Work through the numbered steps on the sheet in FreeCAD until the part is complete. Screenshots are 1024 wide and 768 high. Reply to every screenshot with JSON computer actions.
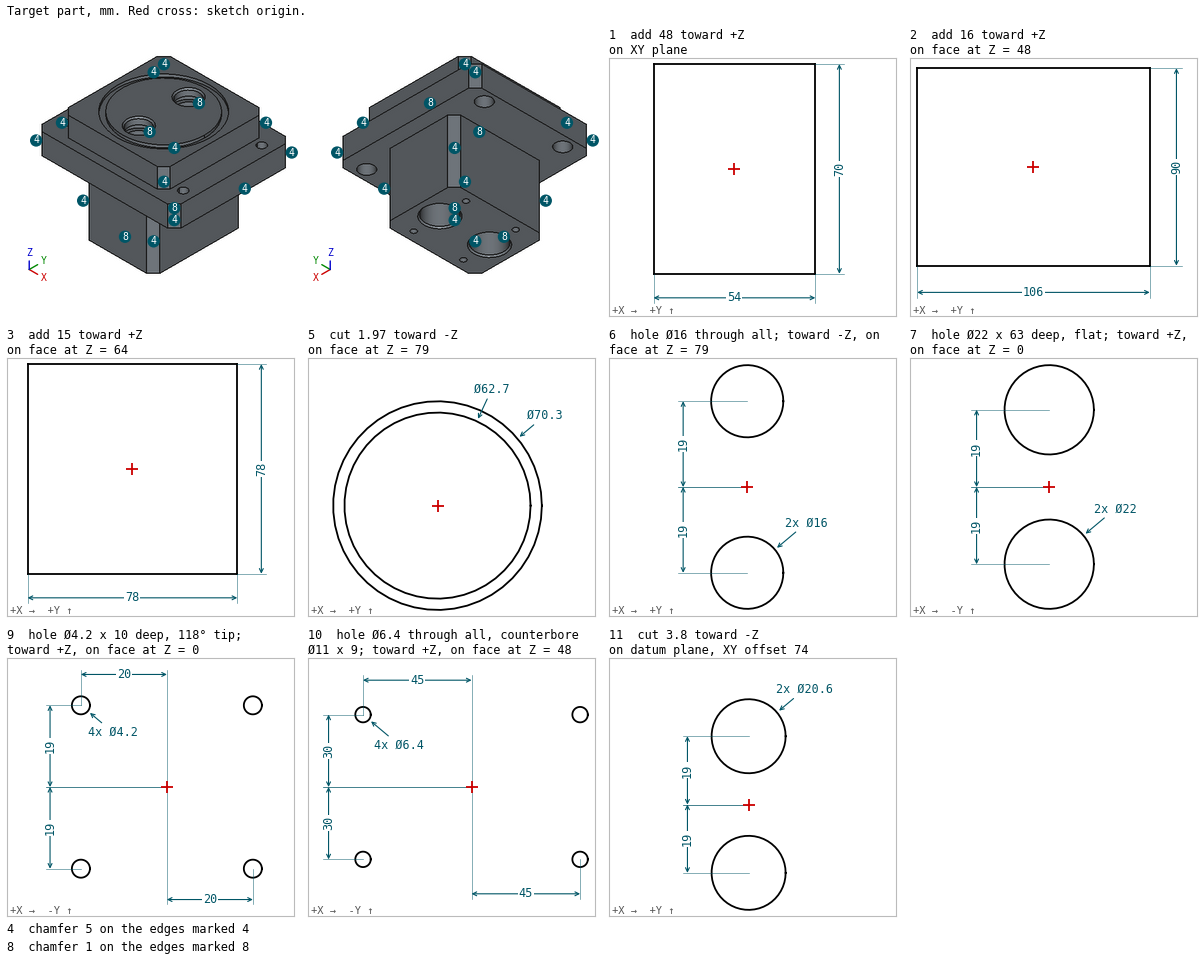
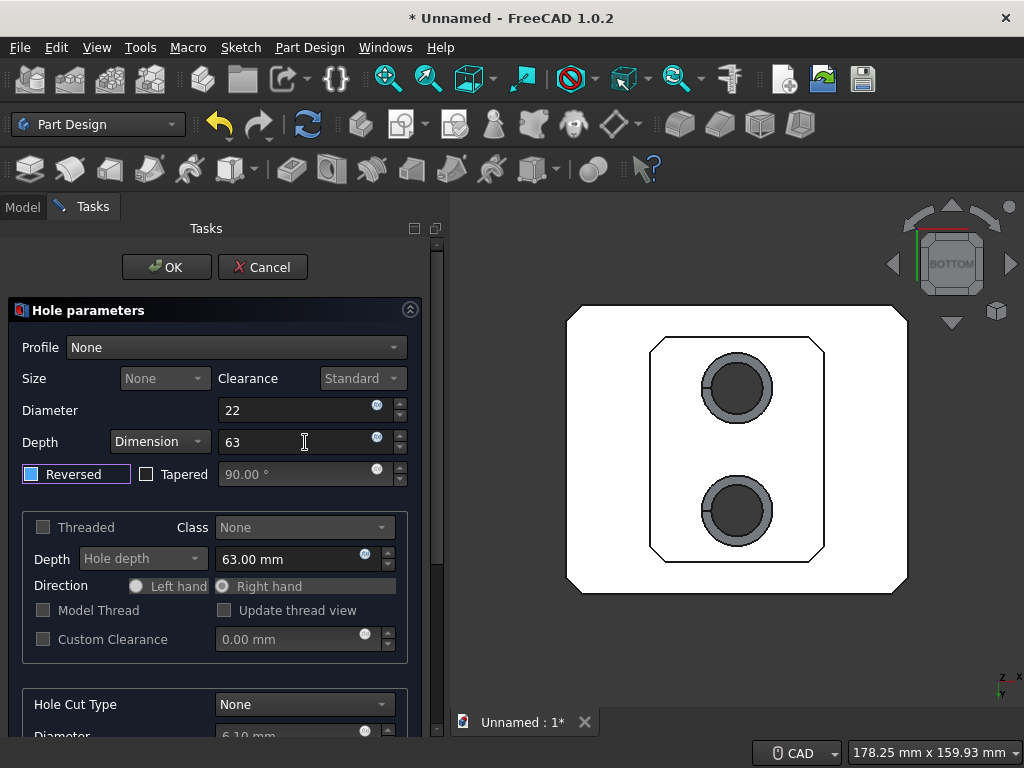
{"action": "scroll", "coordinate": [437, 487], "scroll_direction": "down", "scroll_amount": 4}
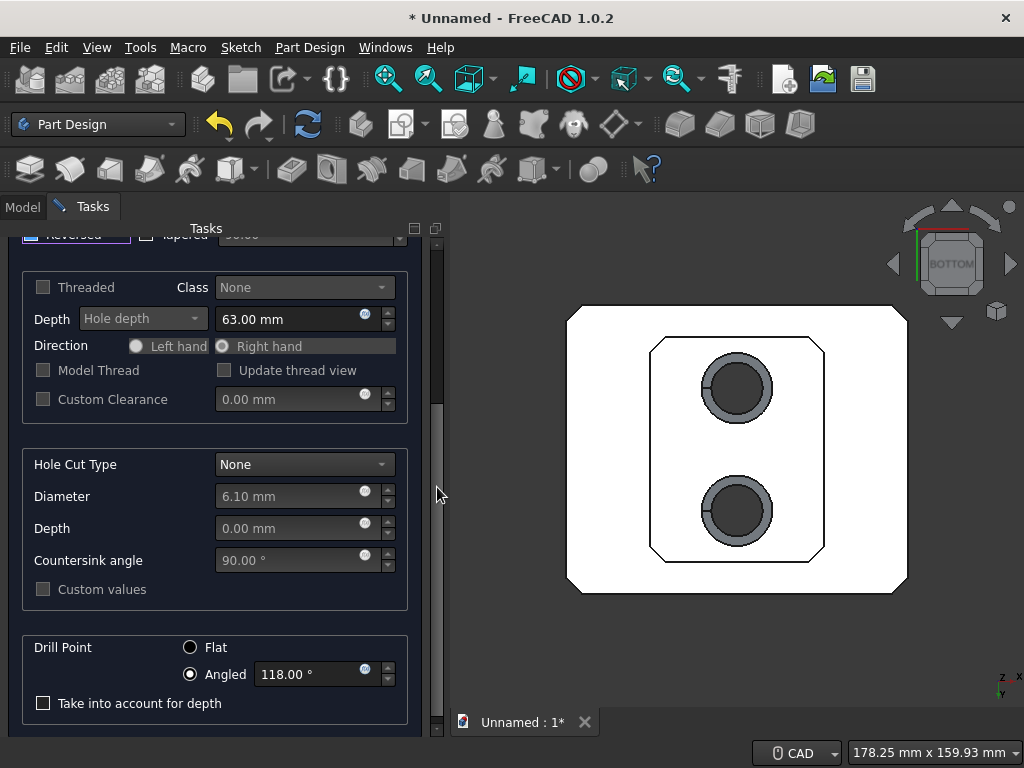
{"action": "left_click", "coordinate": [191, 647]}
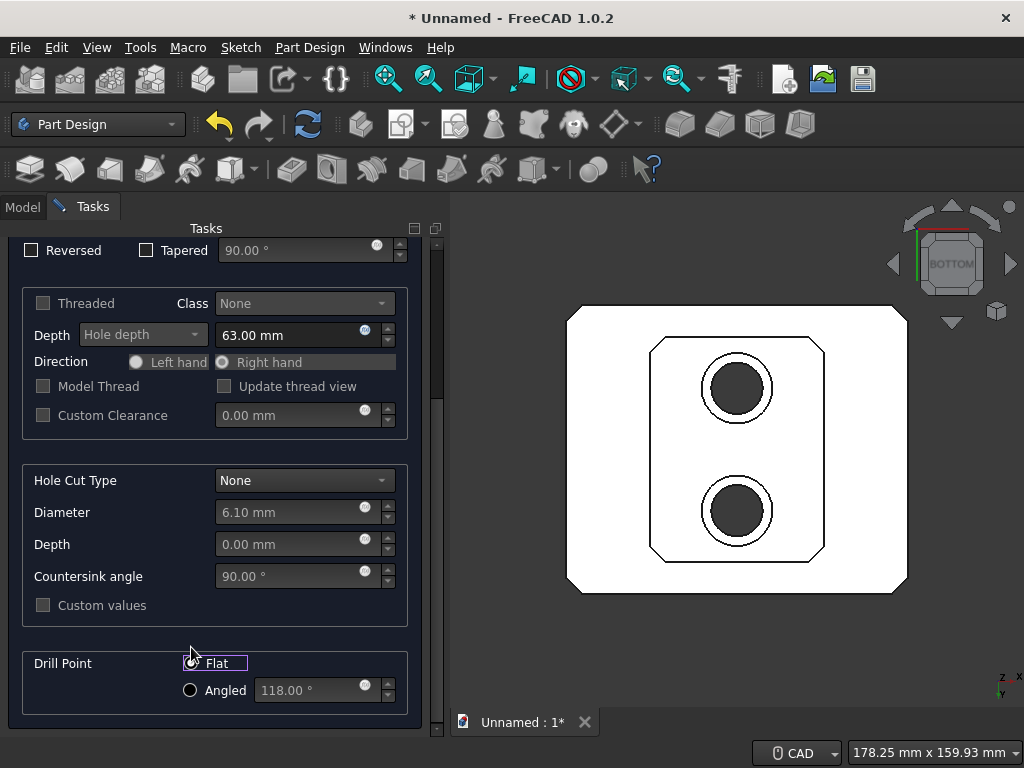
{"action": "scroll", "coordinate": [437, 487], "scroll_direction": "up", "scroll_amount": 5}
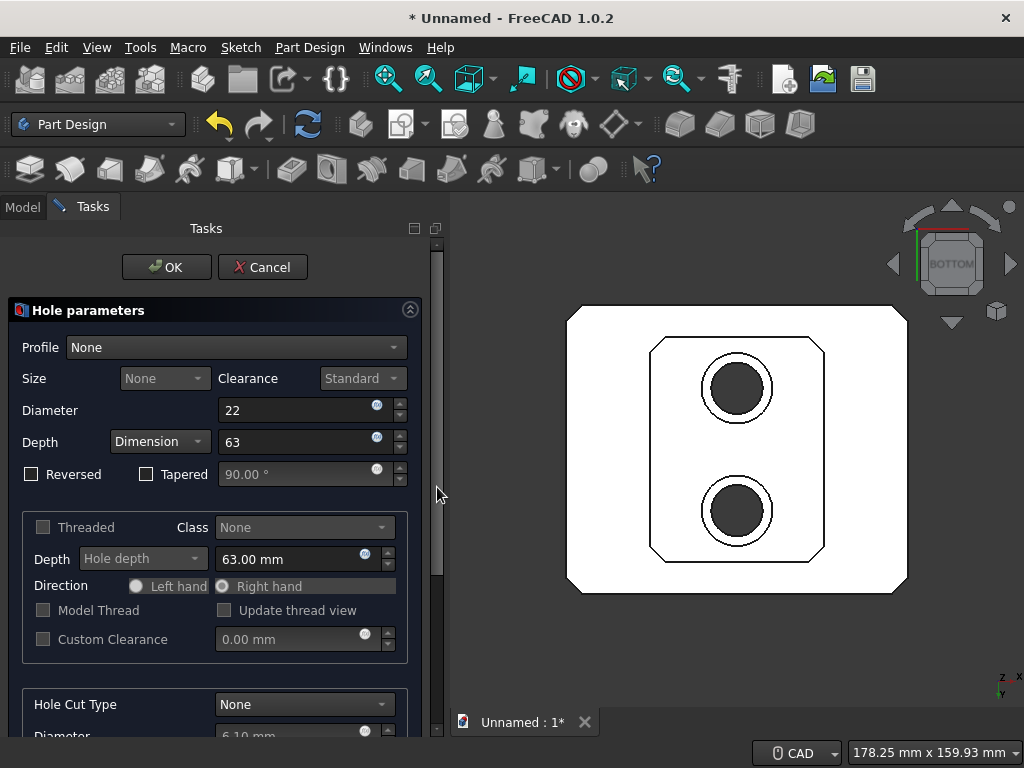
{"action": "left_click", "coordinate": [167, 267]}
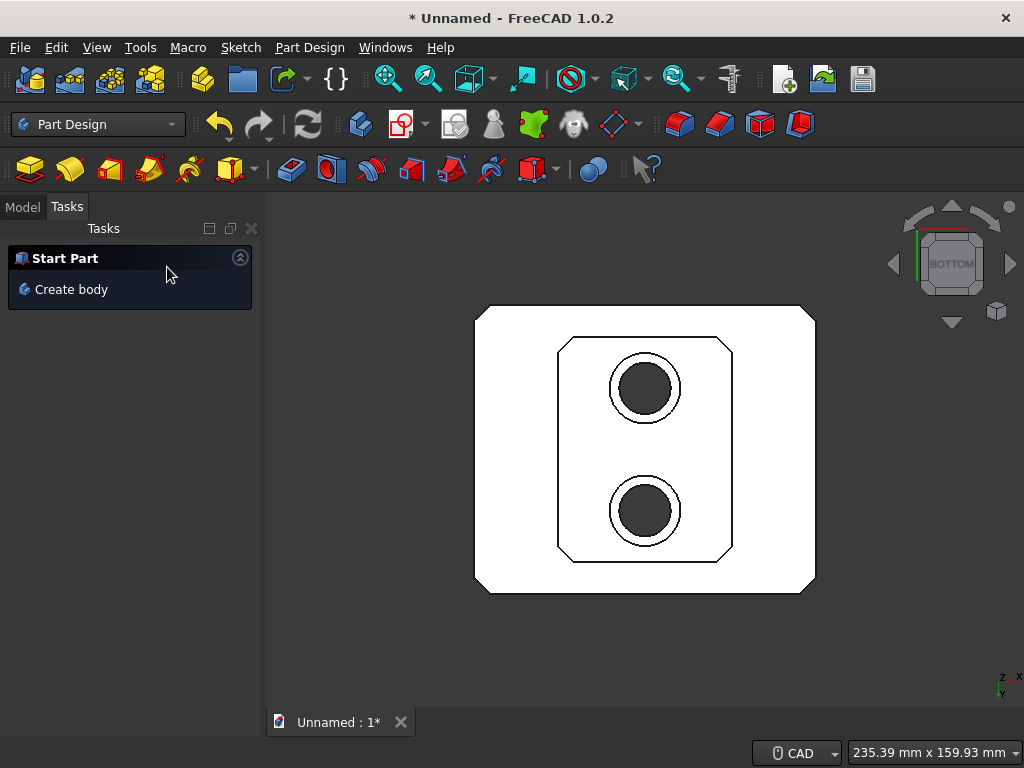
{"action": "left_click", "coordinate": [674, 366]}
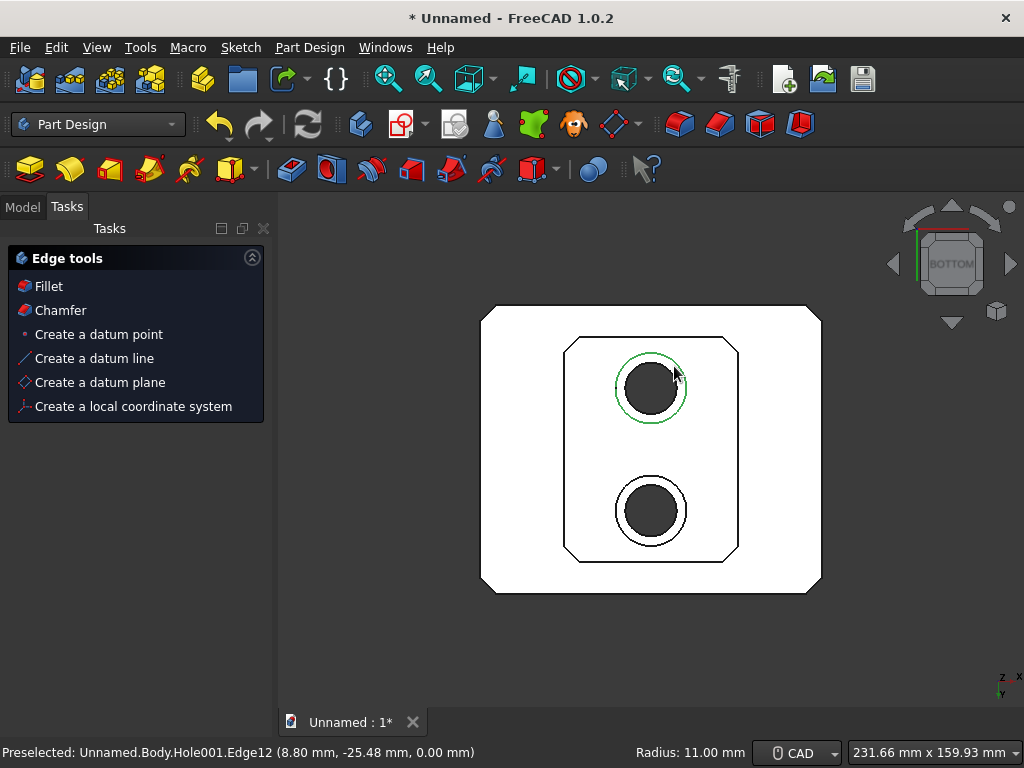
{"action": "left_click", "coordinate": [680, 531], "text": "ctrl"}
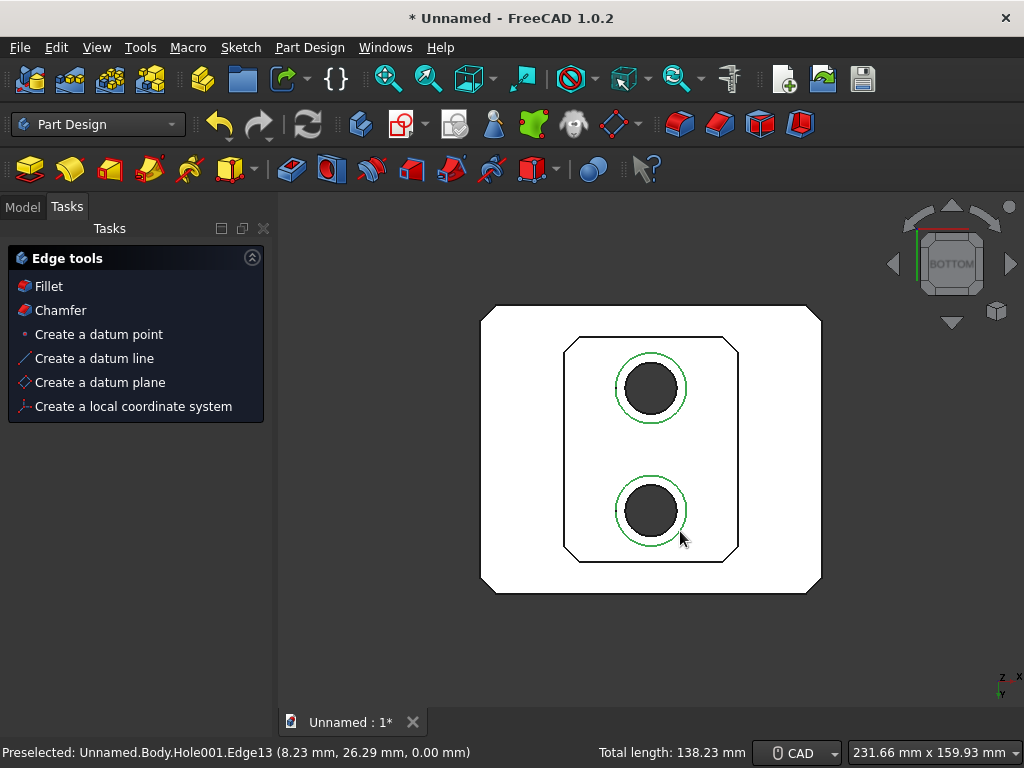
{"action": "key", "text": "0"}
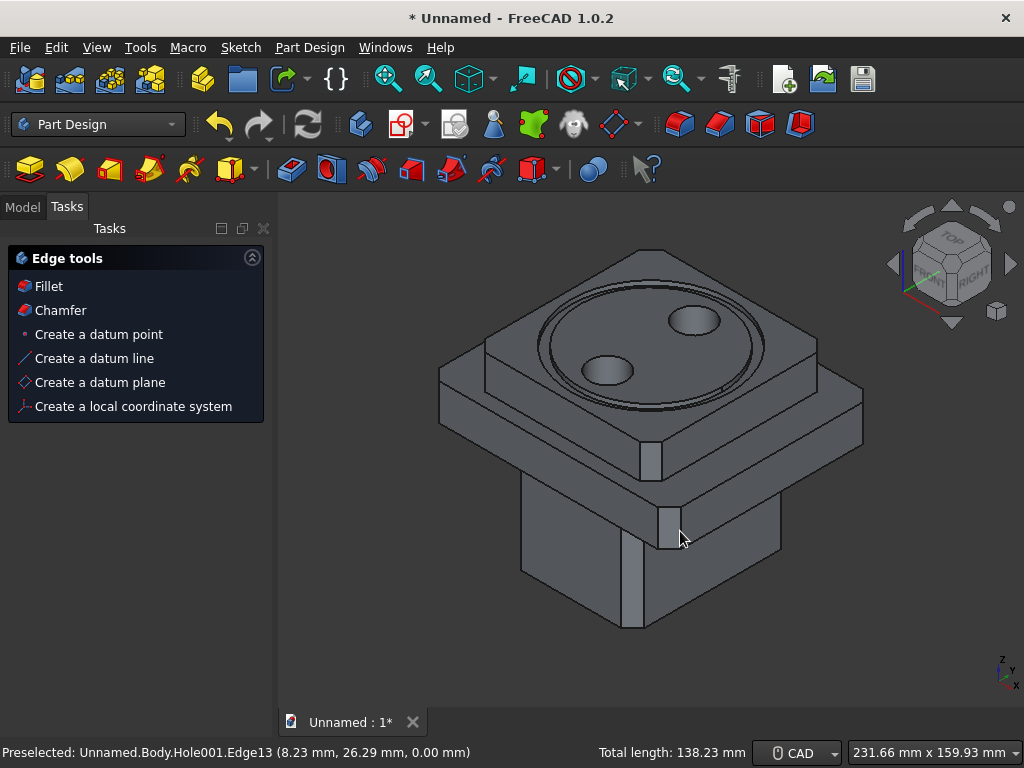
{"action": "left_click", "coordinate": [676, 309], "text": "ctrl"}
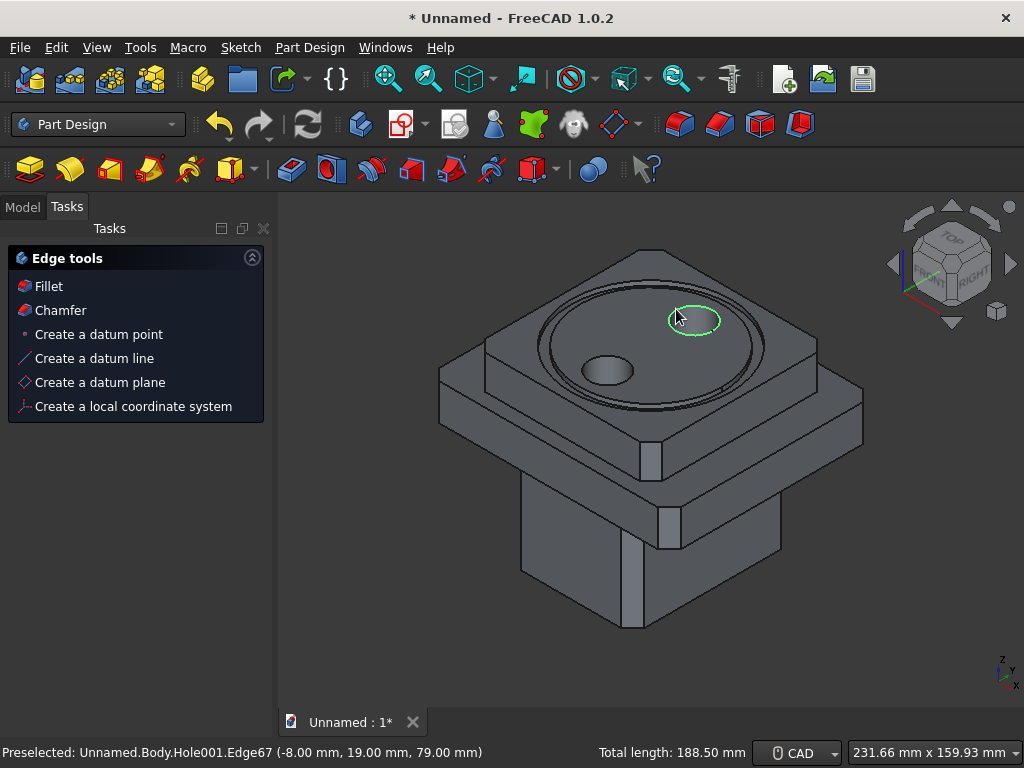
{"action": "left_click", "coordinate": [590, 359], "text": "ctrl"}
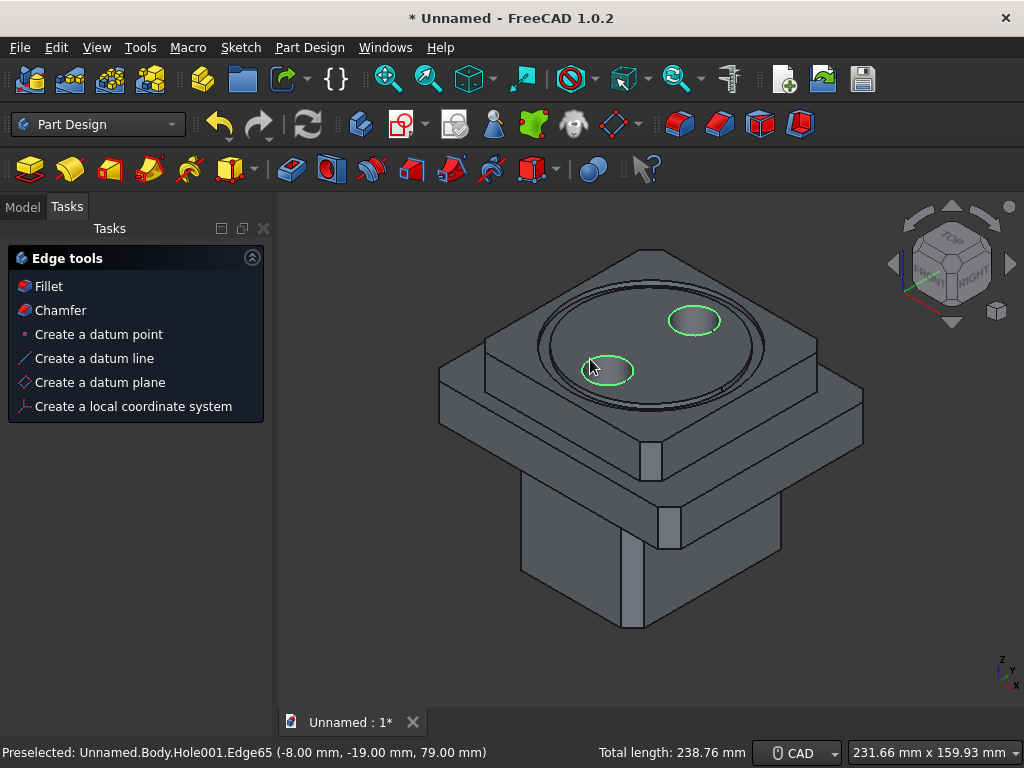
{"action": "left_click", "coordinate": [720, 124]}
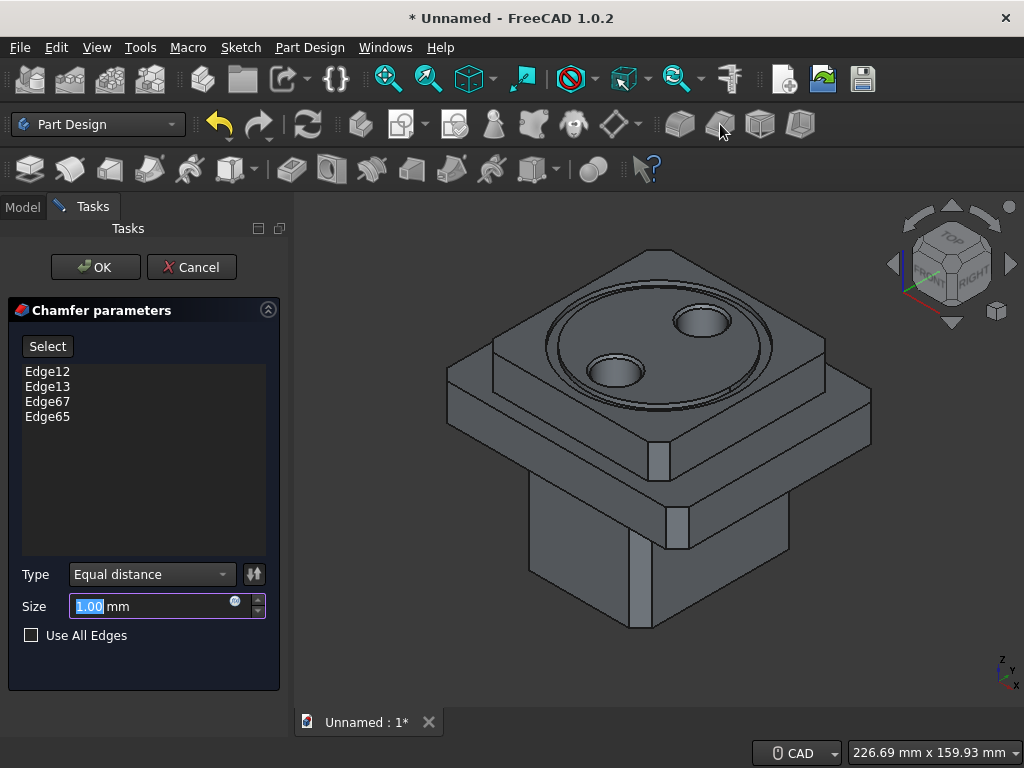
{"action": "type", "text": "1"}
{"action": "key", "text": "Tab"}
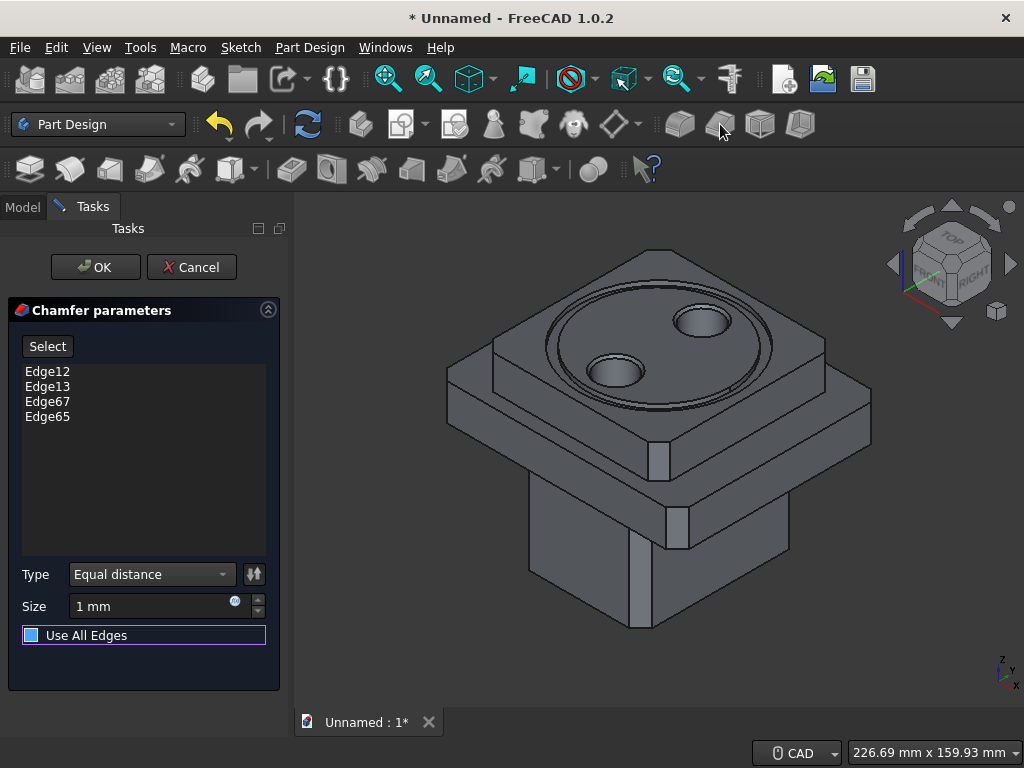
{"action": "left_click", "coordinate": [96, 267]}